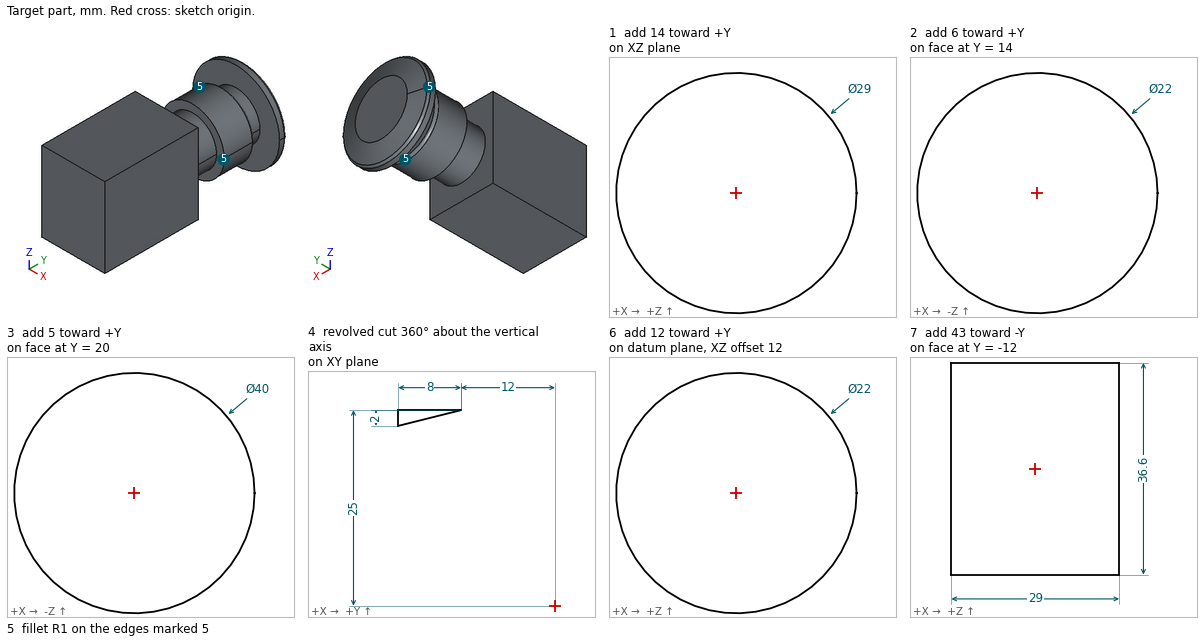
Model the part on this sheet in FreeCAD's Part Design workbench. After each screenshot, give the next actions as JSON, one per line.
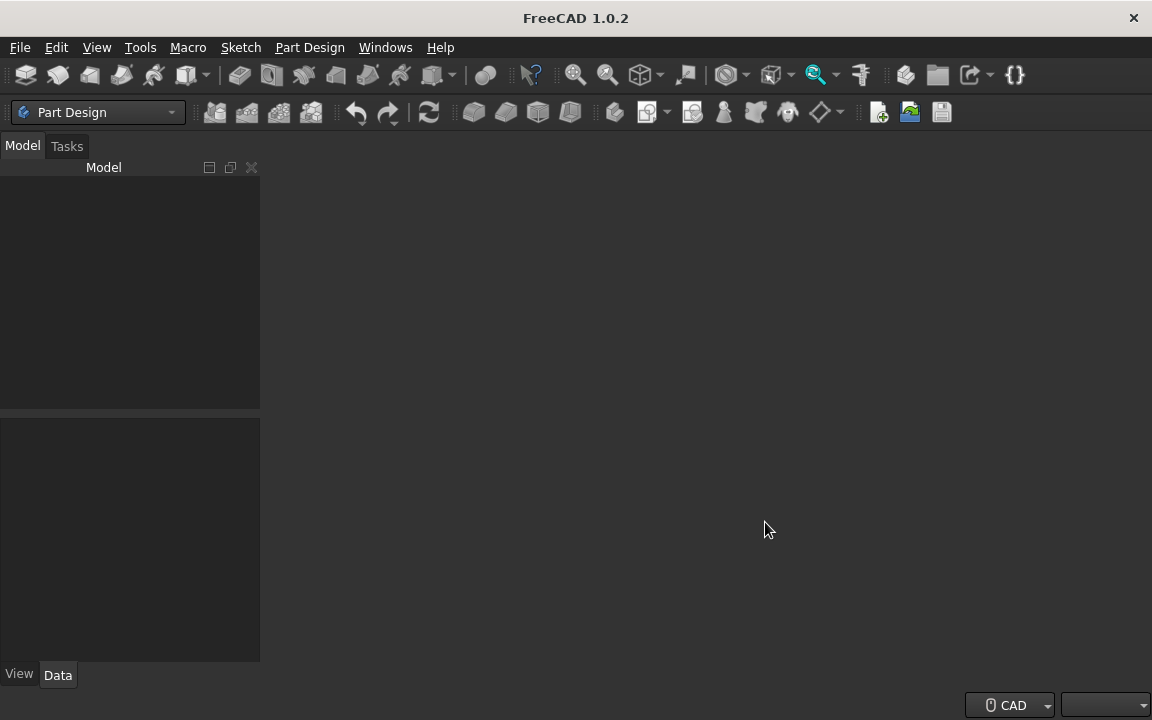
{"action": "key", "text": "ctrl+n"}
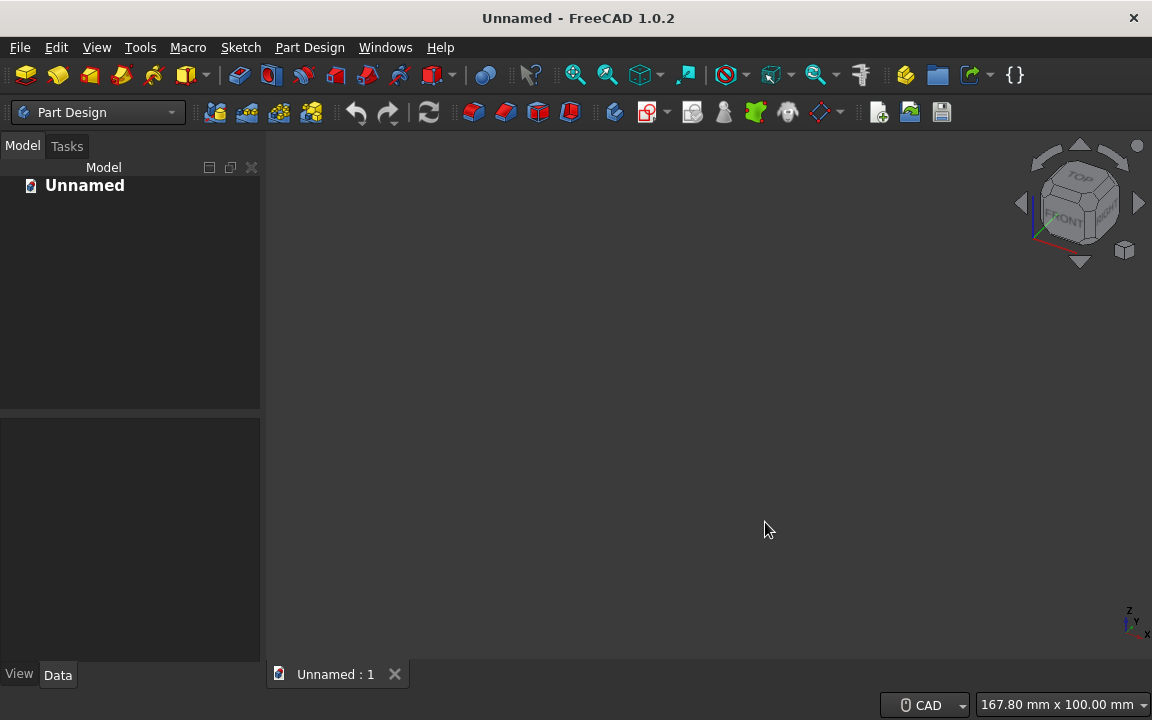
{"action": "left_click", "coordinate": [648, 112]}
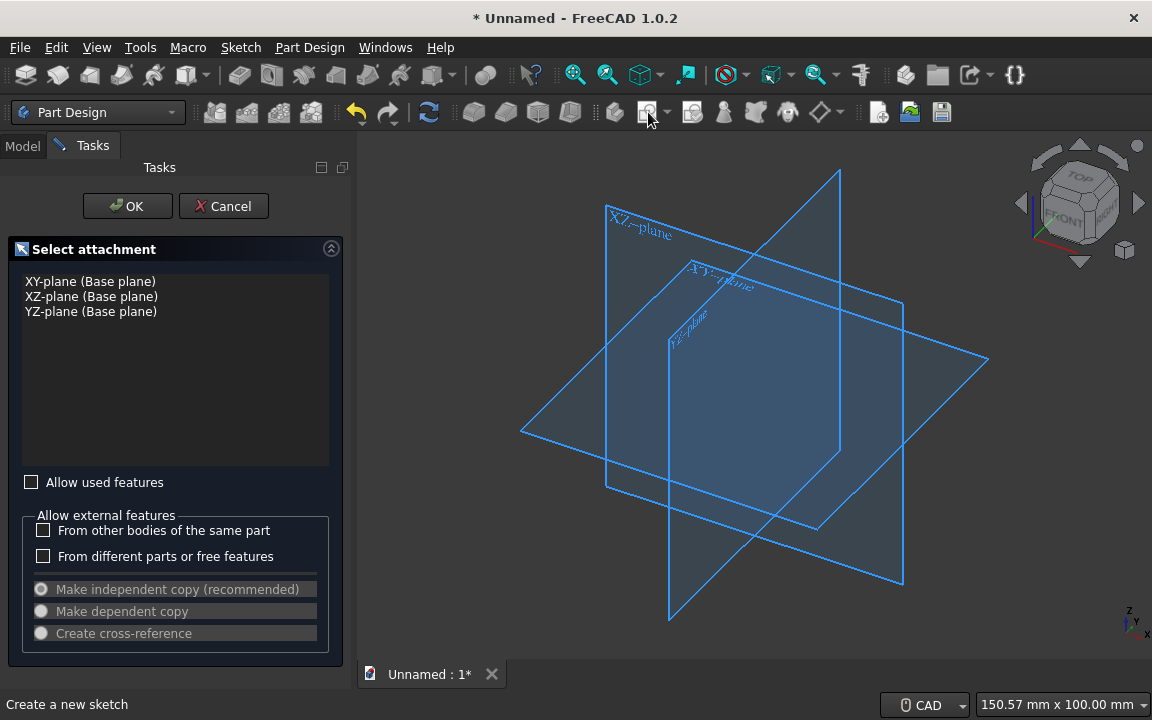
{"action": "left_click", "coordinate": [82, 296]}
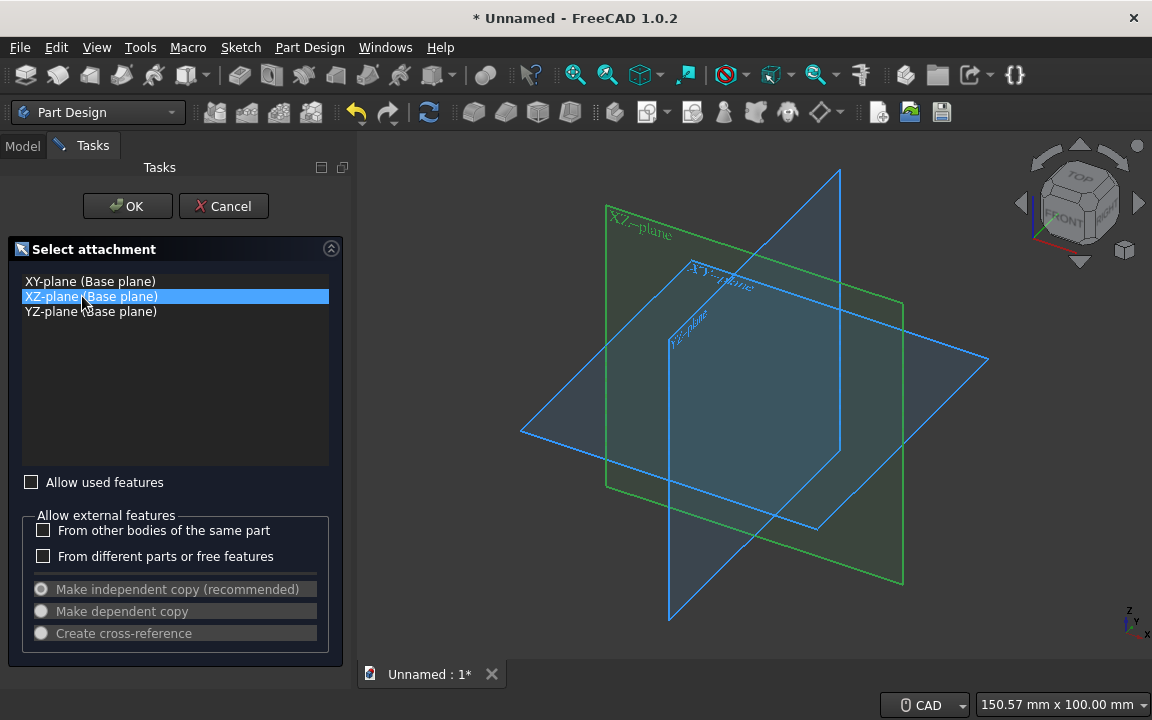
{"action": "left_click", "coordinate": [128, 206]}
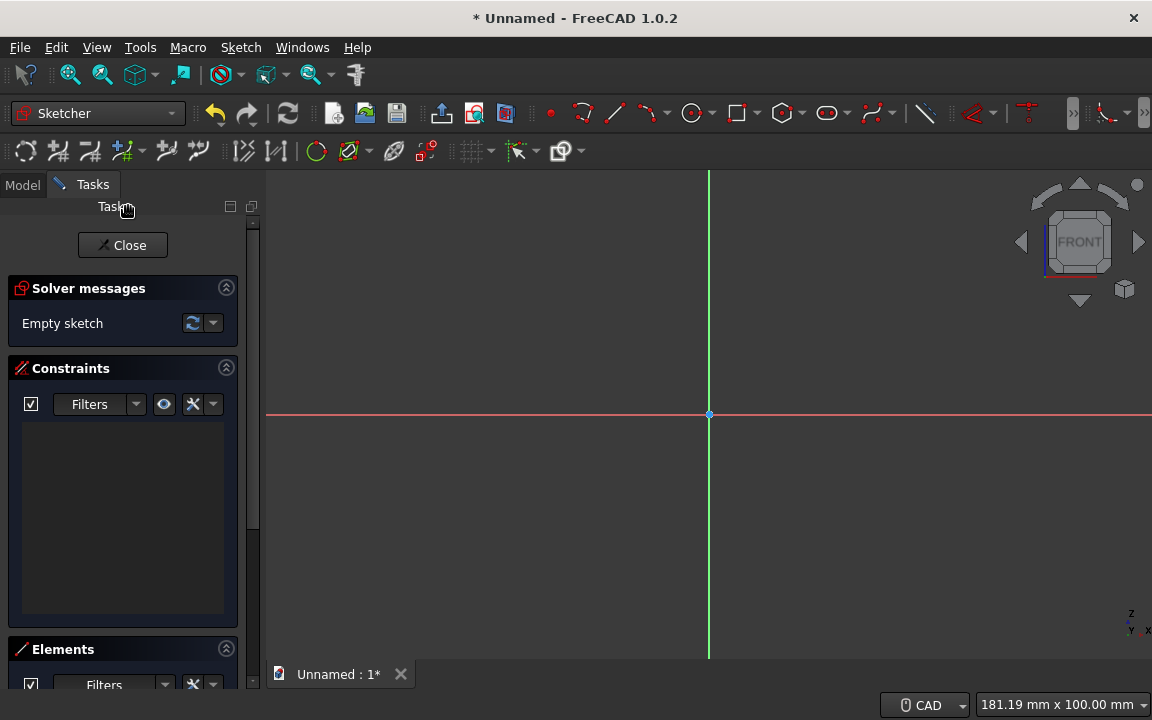
{"action": "scroll", "coordinate": [765, 414], "scroll_direction": "up", "scroll_amount": 4}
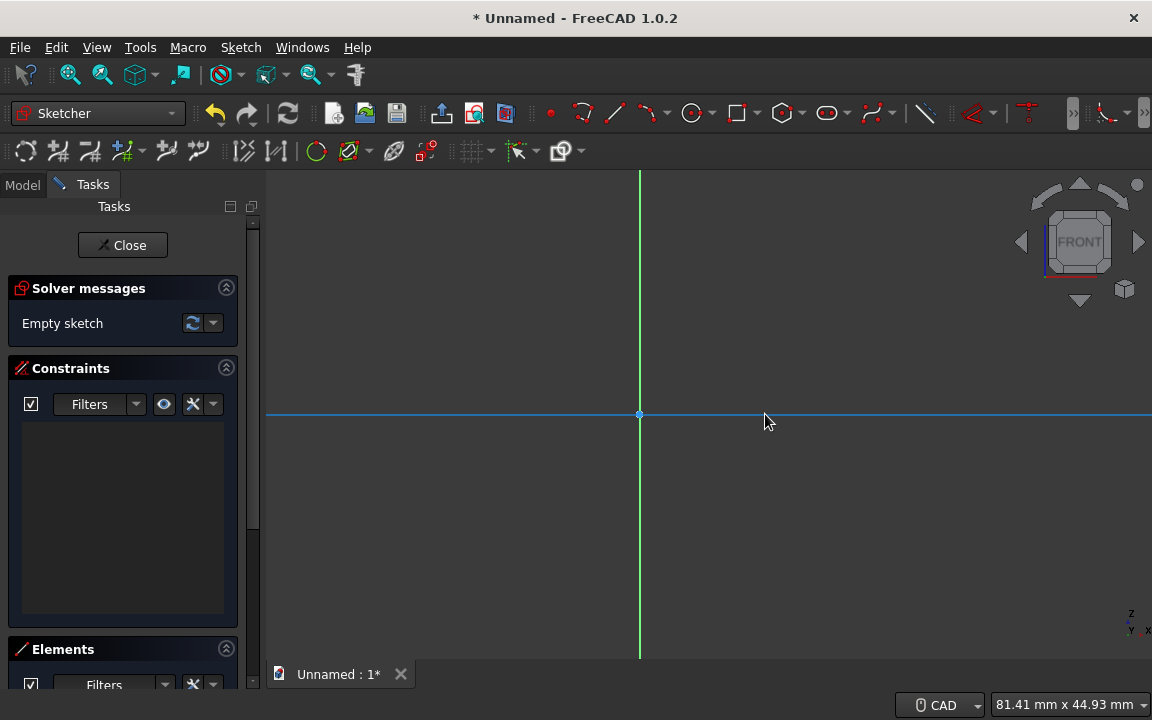
{"action": "left_click", "coordinate": [692, 114]}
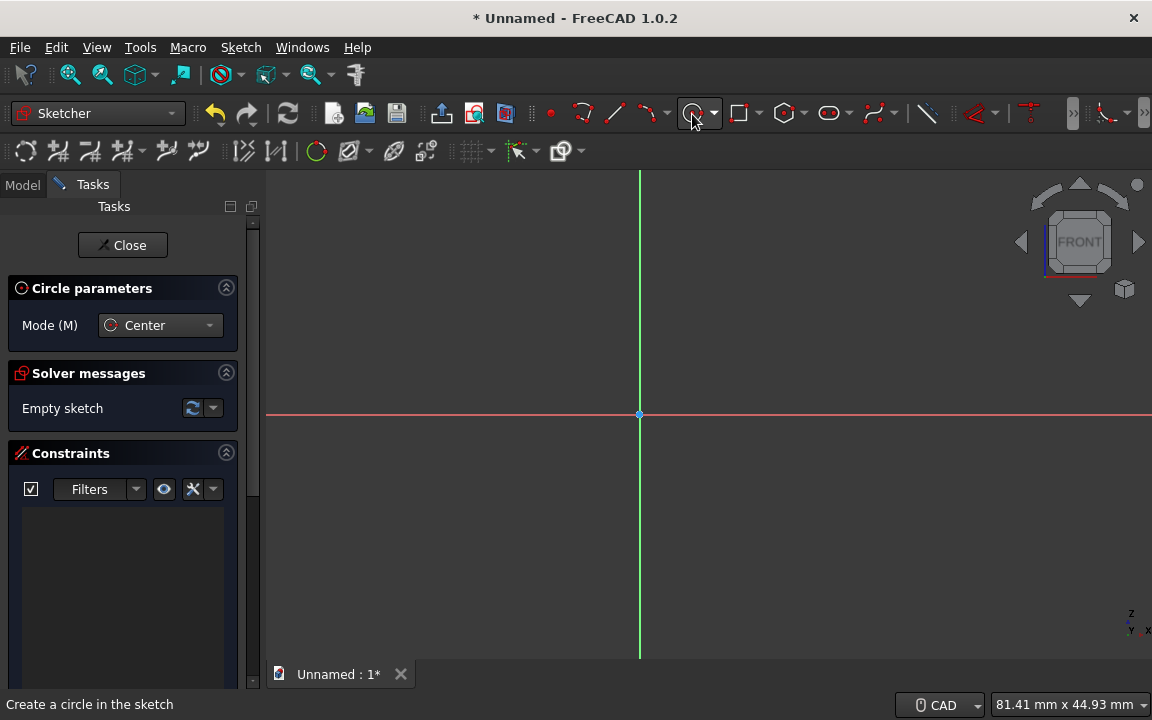
{"action": "left_click", "coordinate": [640, 414]}
{"action": "left_click", "coordinate": [751, 303]}
{"action": "key", "text": "Escape"}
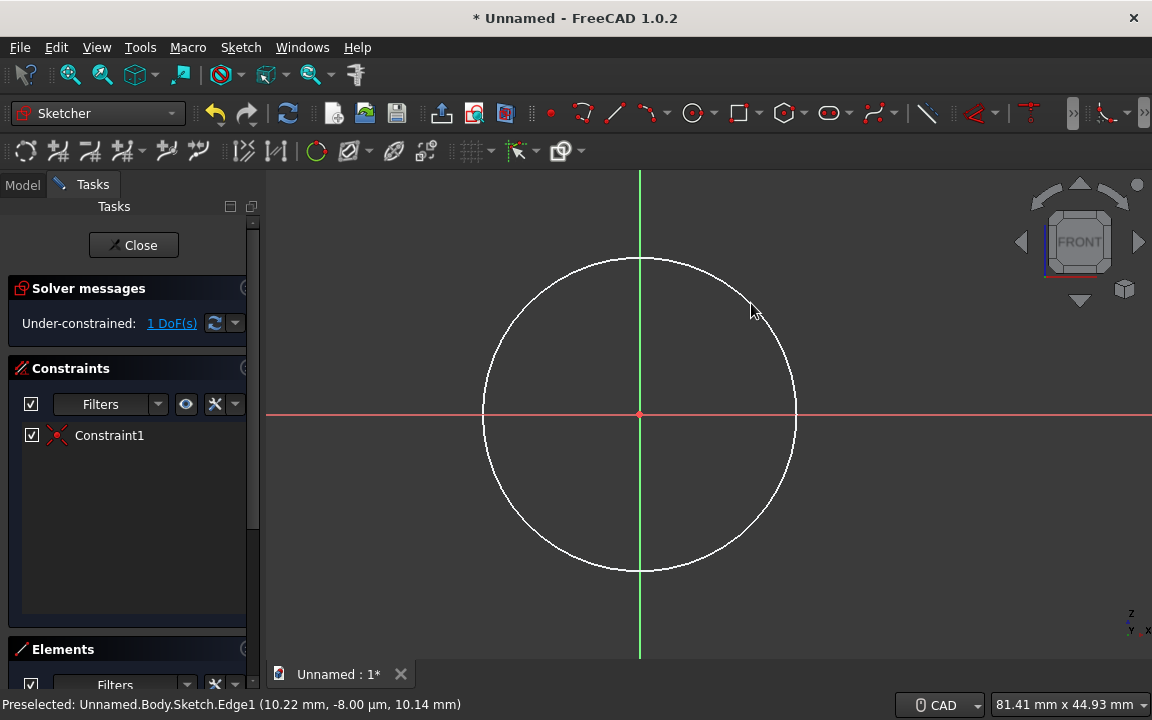
{"action": "left_click", "coordinate": [750, 303]}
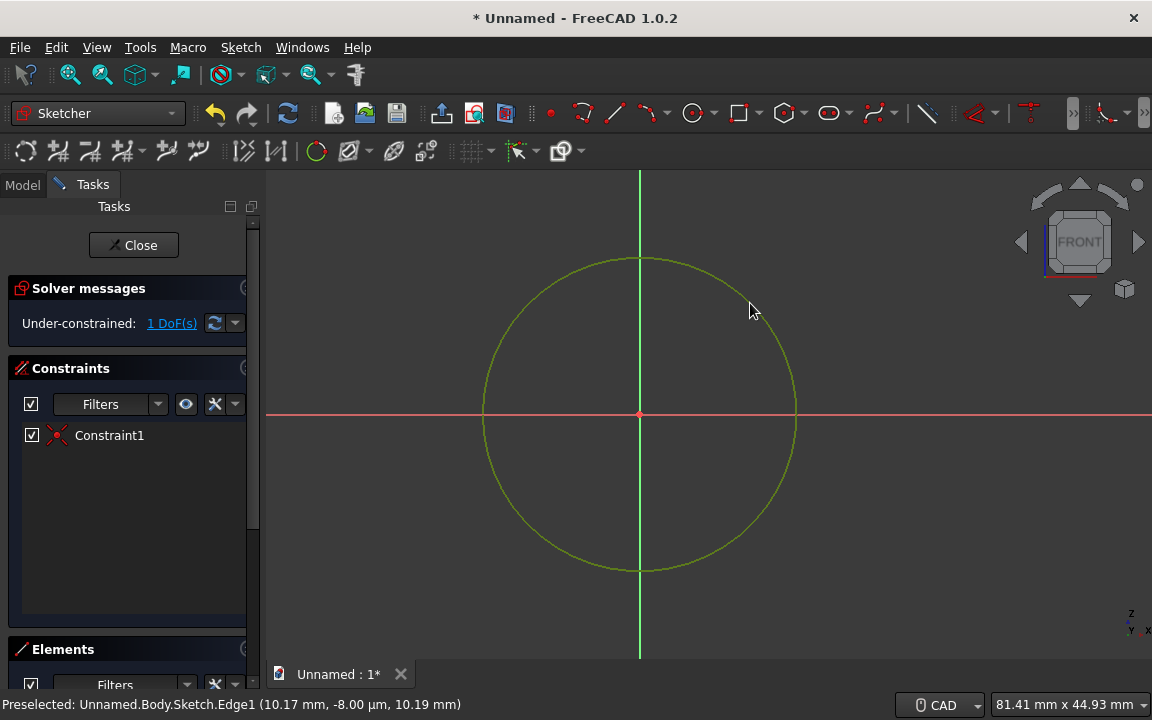
{"action": "key", "text": "k o"}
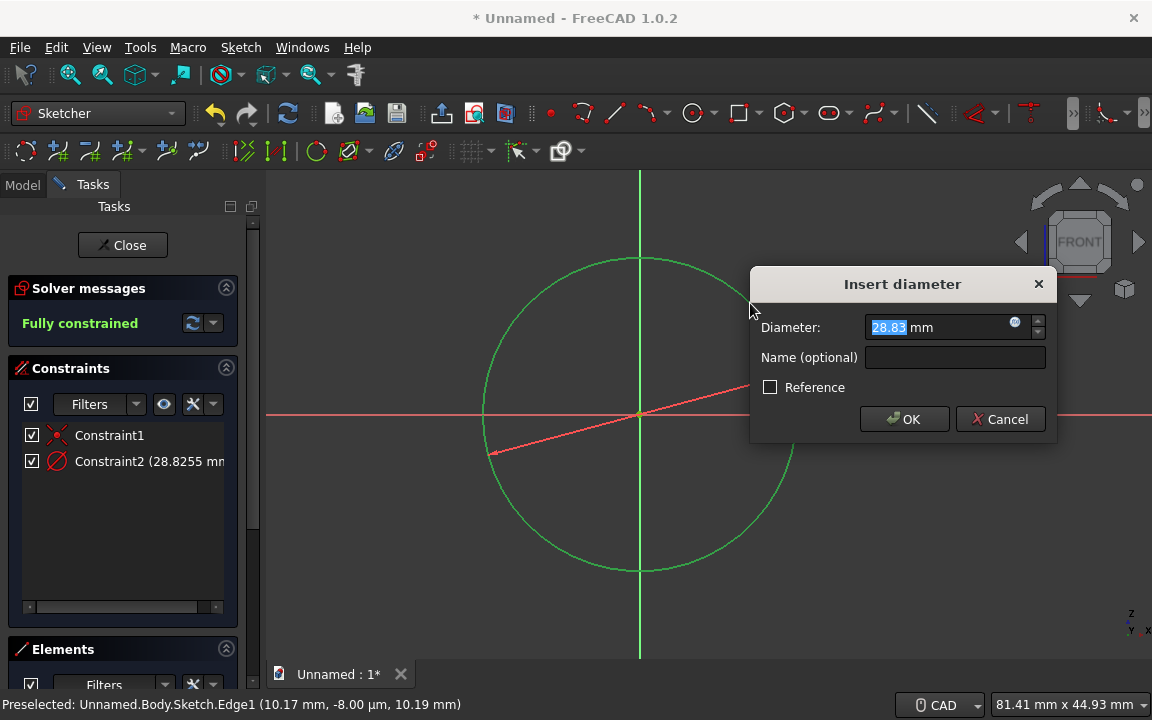
{"action": "type", "text": "29"}
{"action": "key", "text": "Return"}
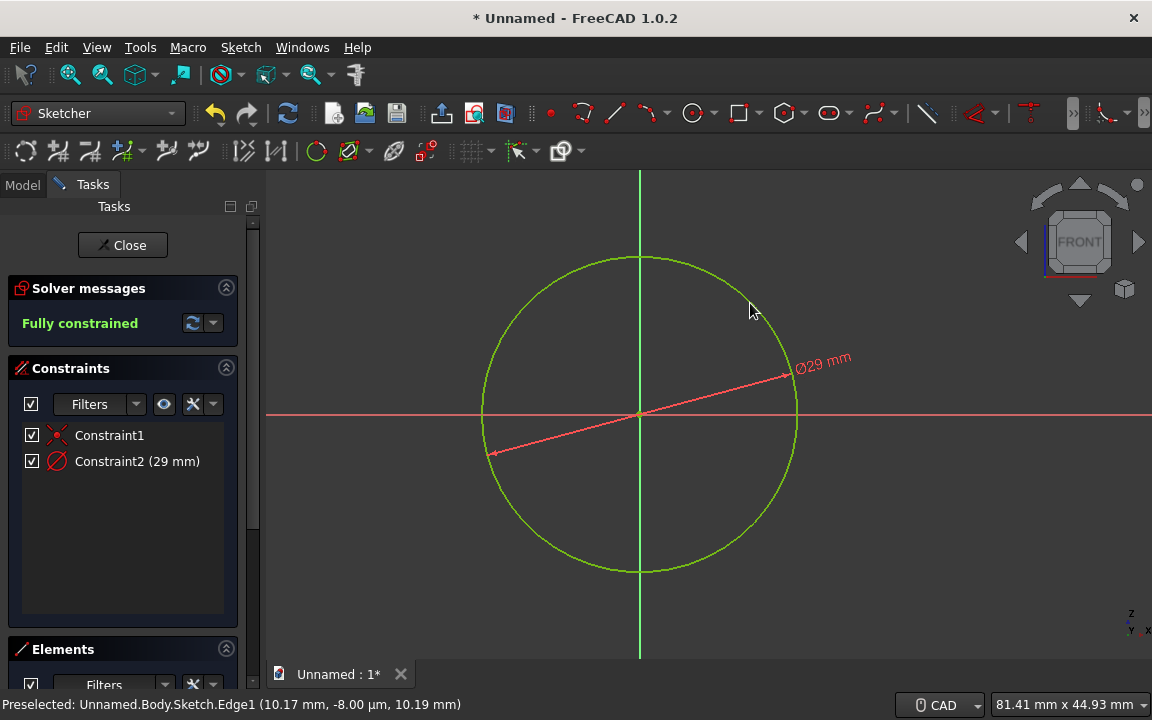
{"action": "left_click", "coordinate": [123, 245]}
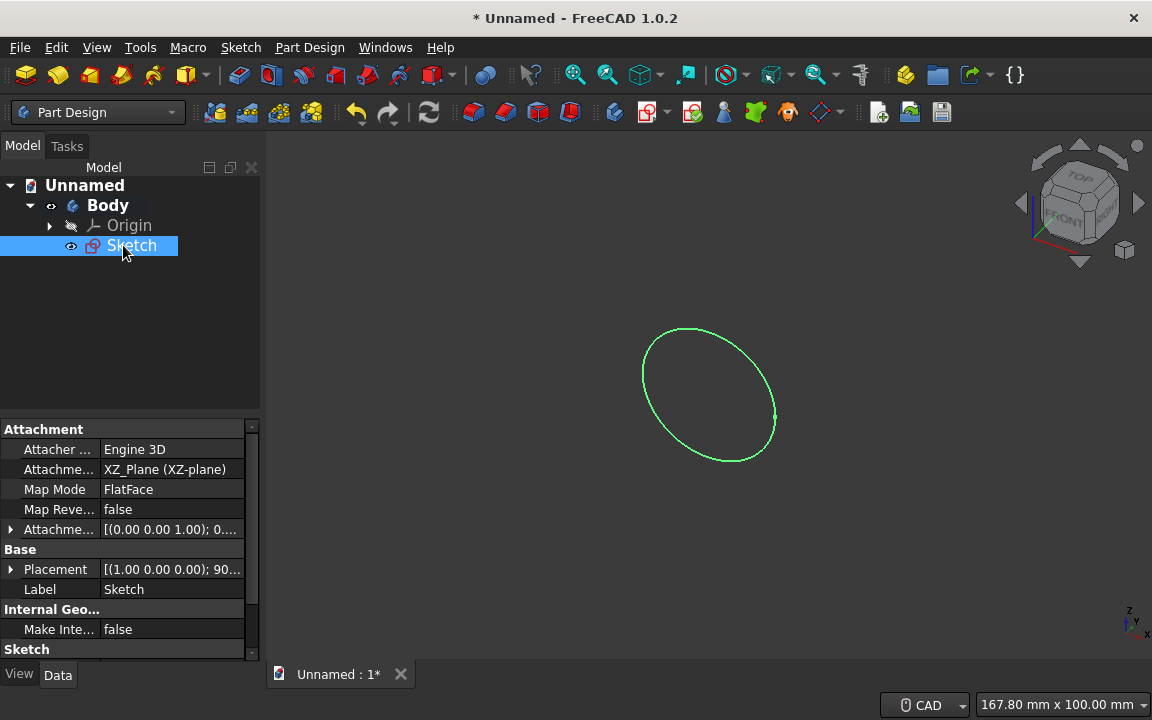
{"action": "left_click", "coordinate": [26, 76]}